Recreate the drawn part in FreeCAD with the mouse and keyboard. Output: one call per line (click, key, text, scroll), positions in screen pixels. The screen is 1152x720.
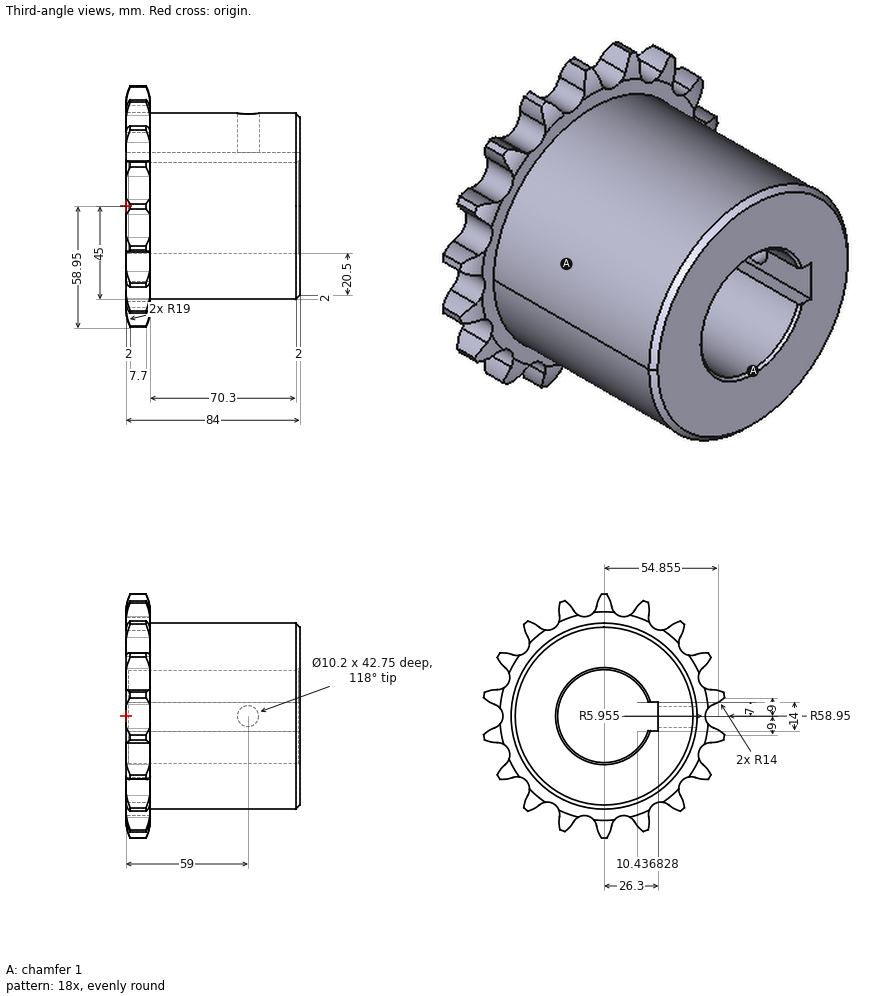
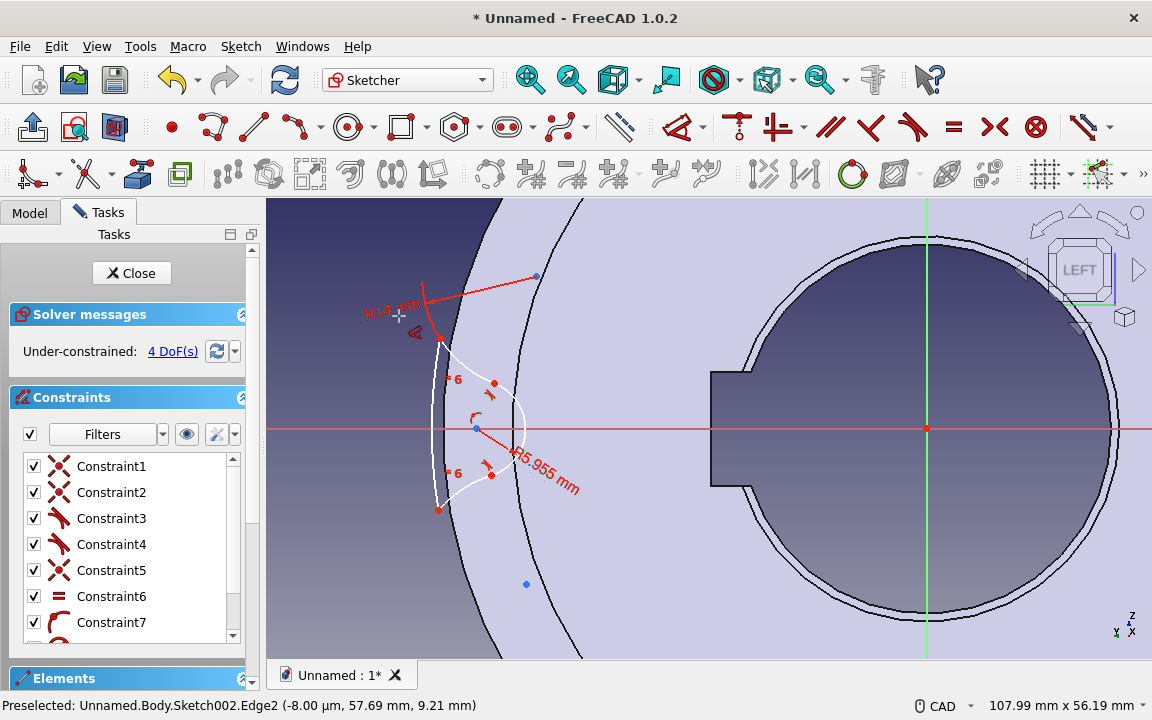
click(433, 390)
click(401, 387)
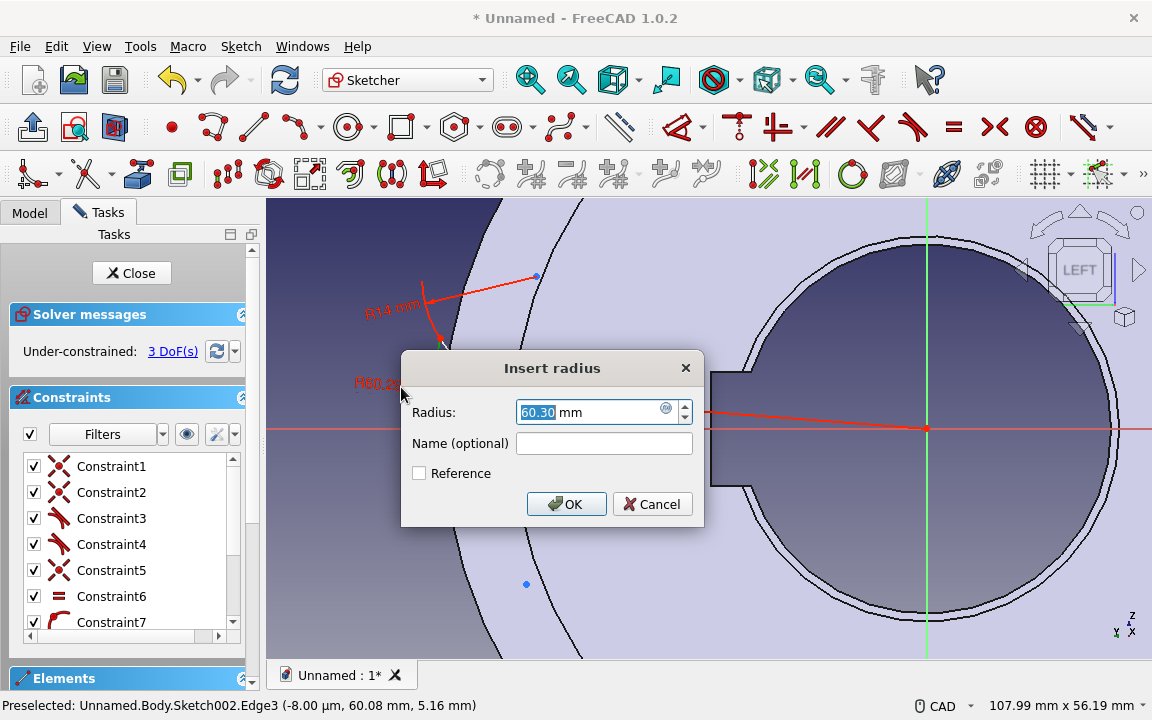
text(58.95)
key(Return)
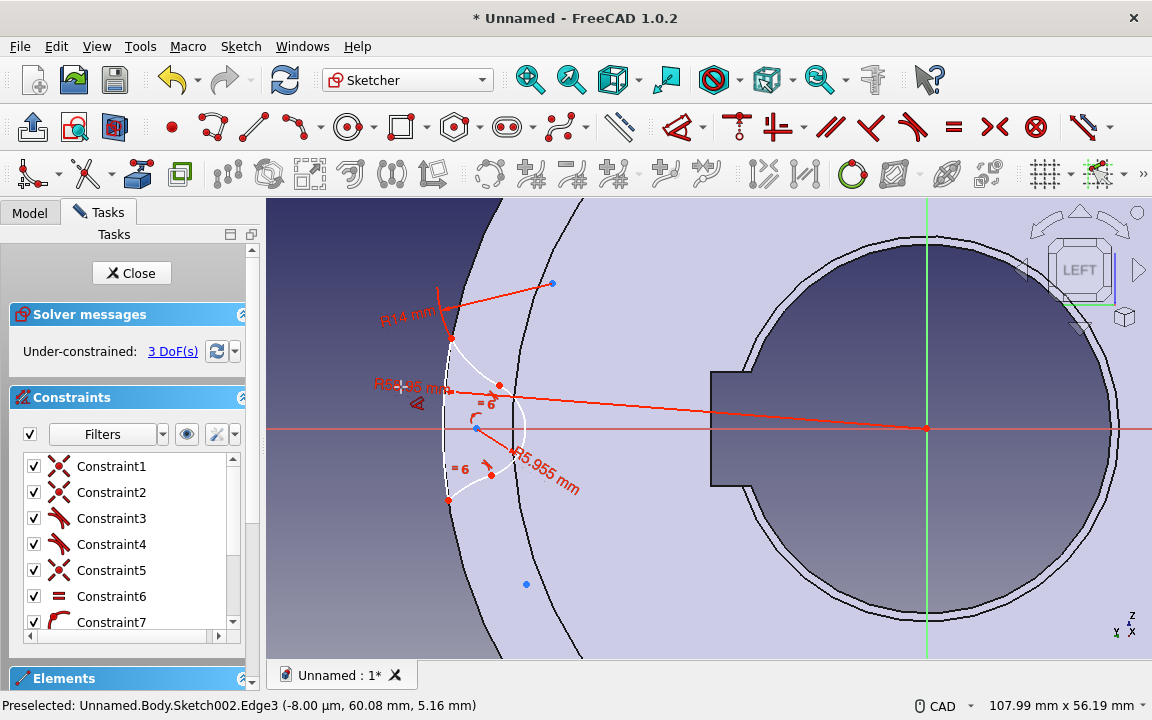
click(451, 339)
click(961, 384)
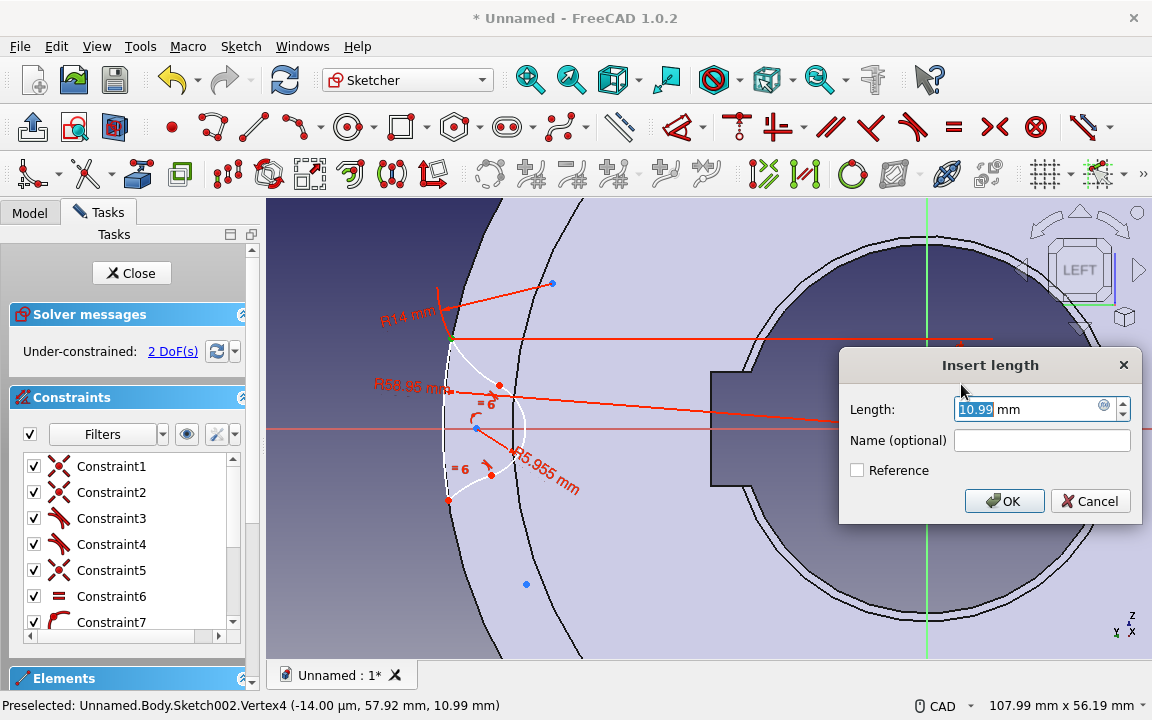
text(9)
key(Return)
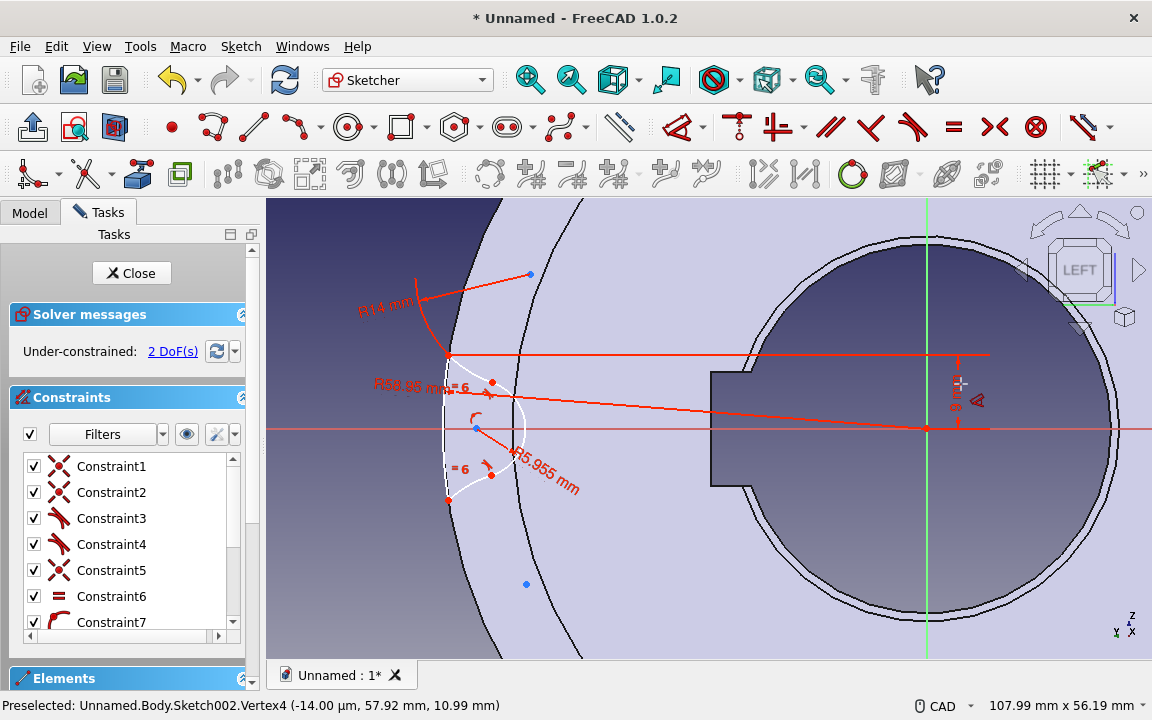
click(448, 501)
click(961, 465)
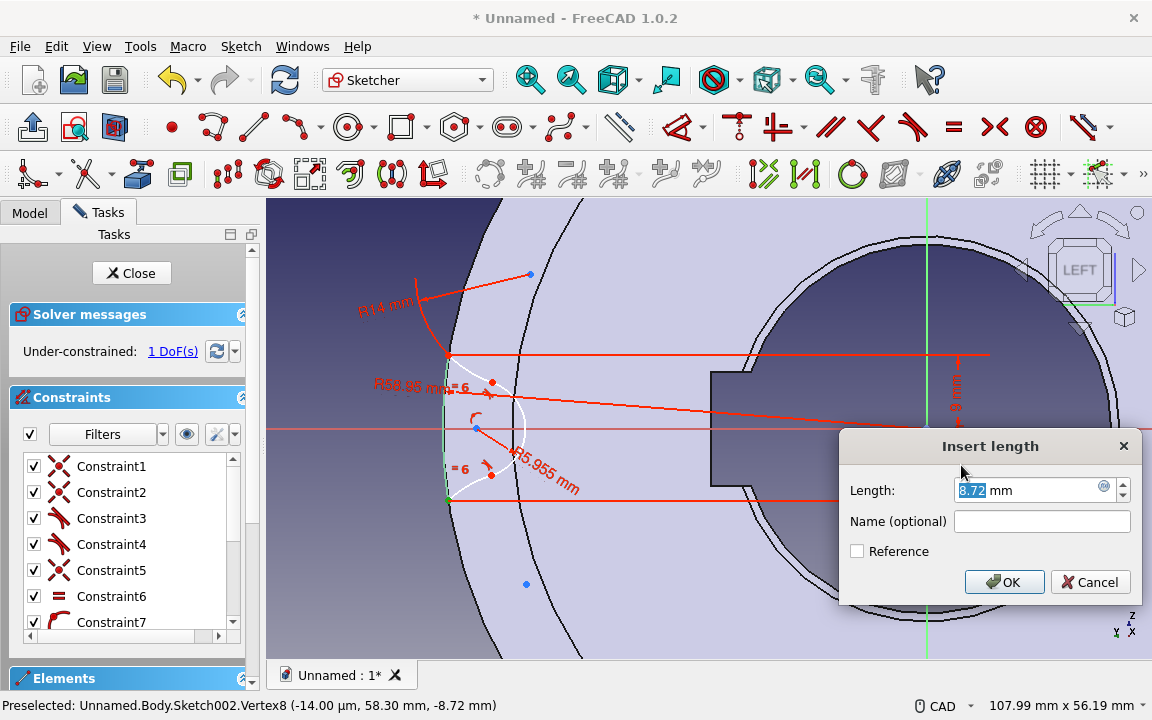
text(9)
key(Return)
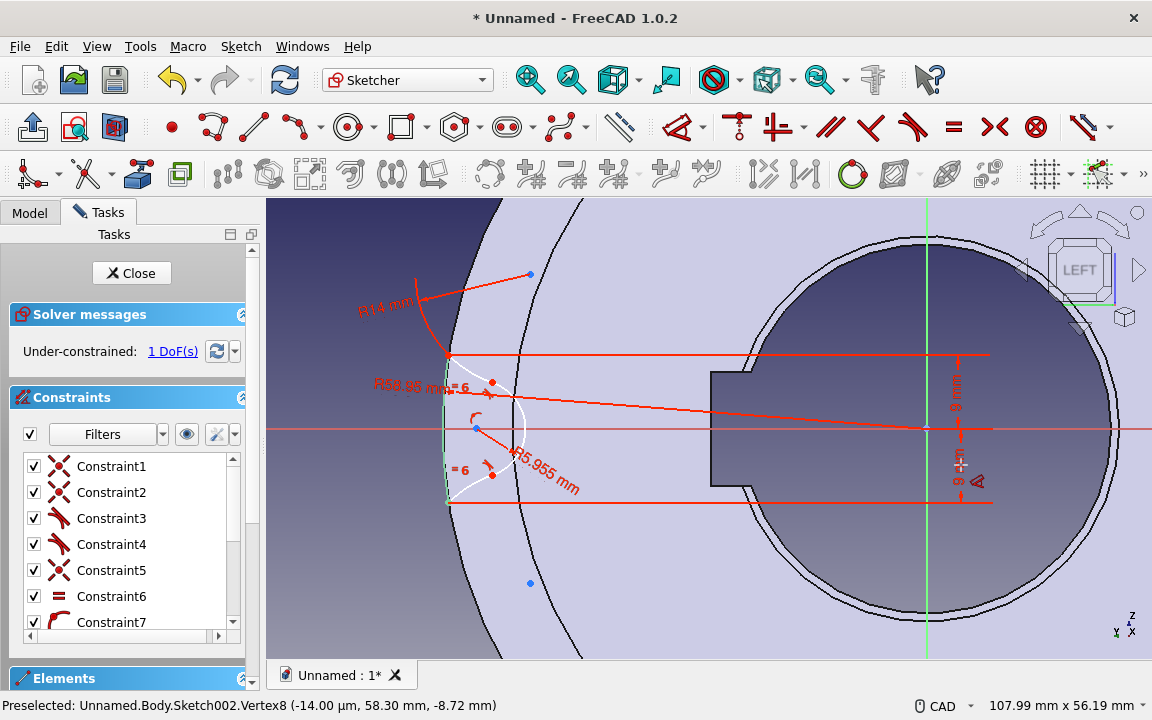
click(477, 429)
click(702, 463)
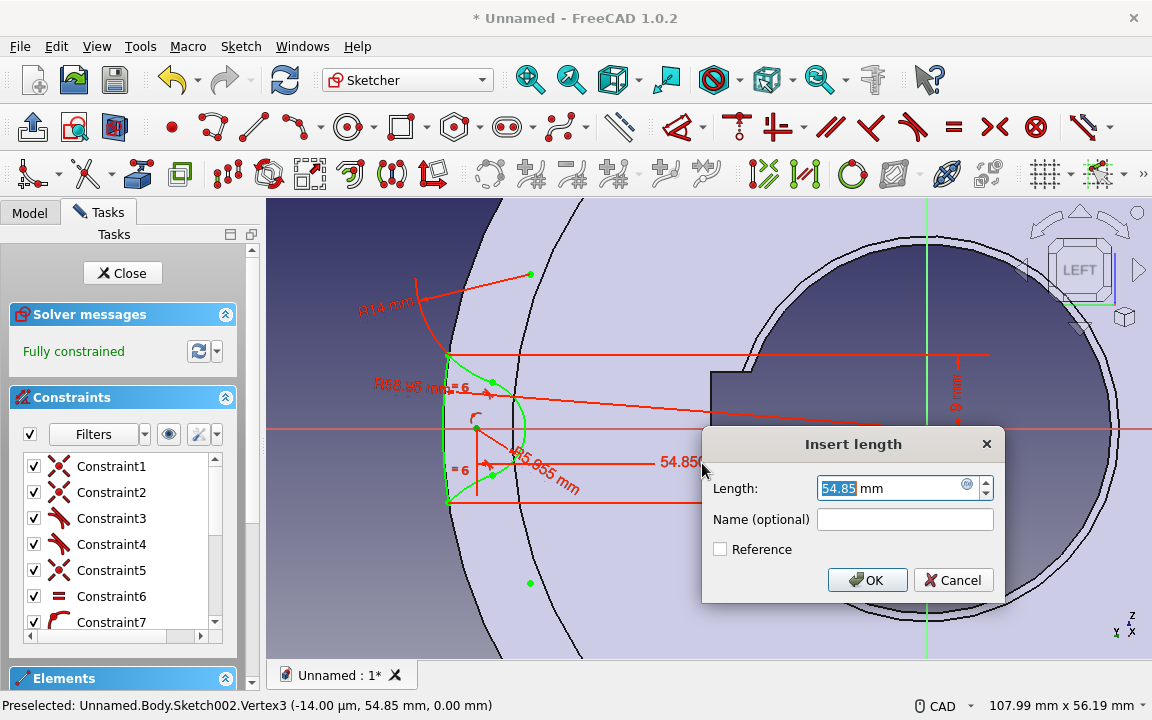
text(54.855)
key(Return)
key(Escape)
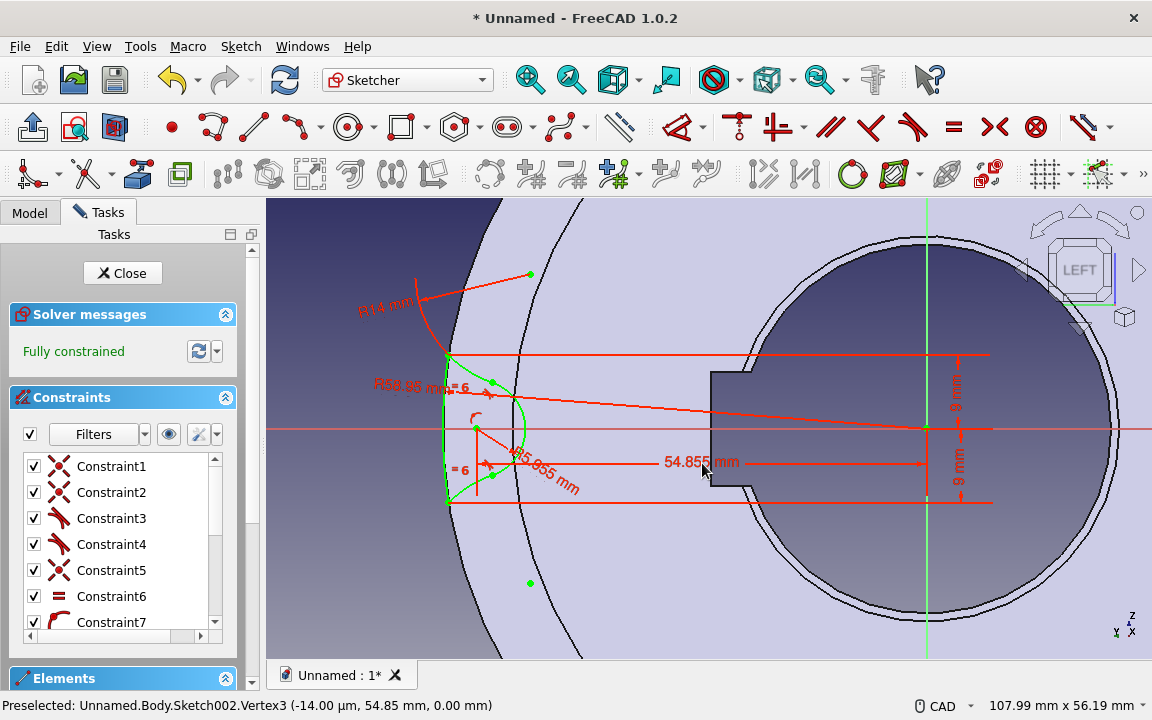
click(123, 273)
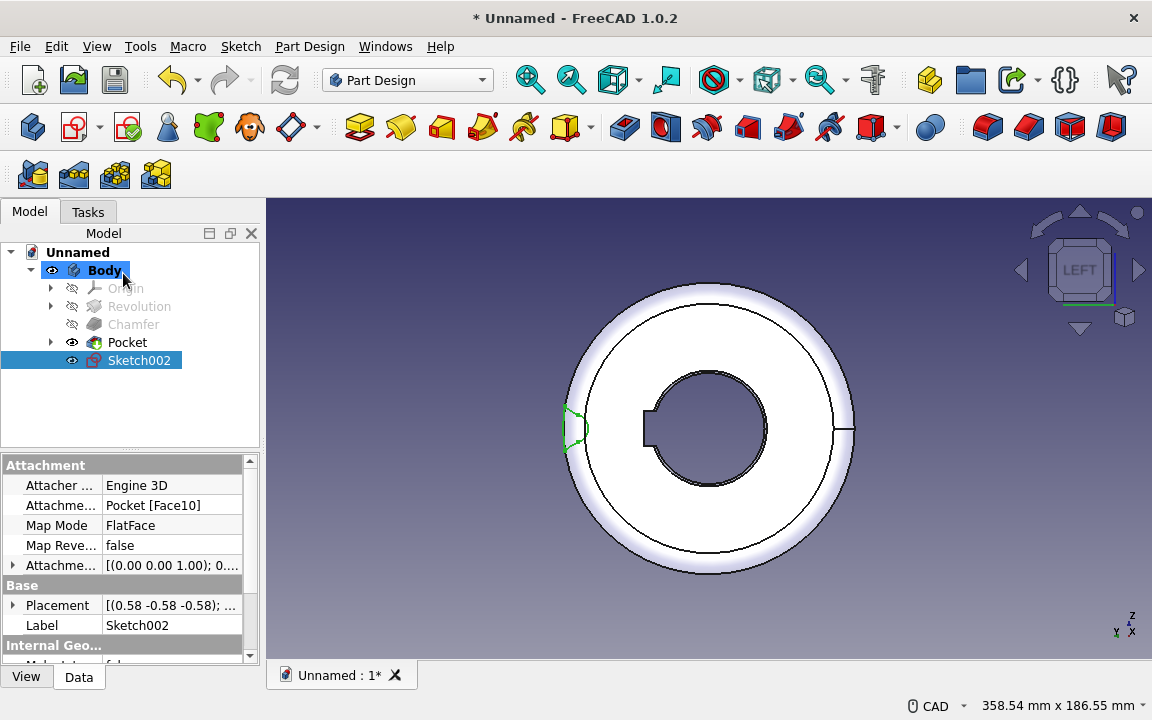
click(625, 128)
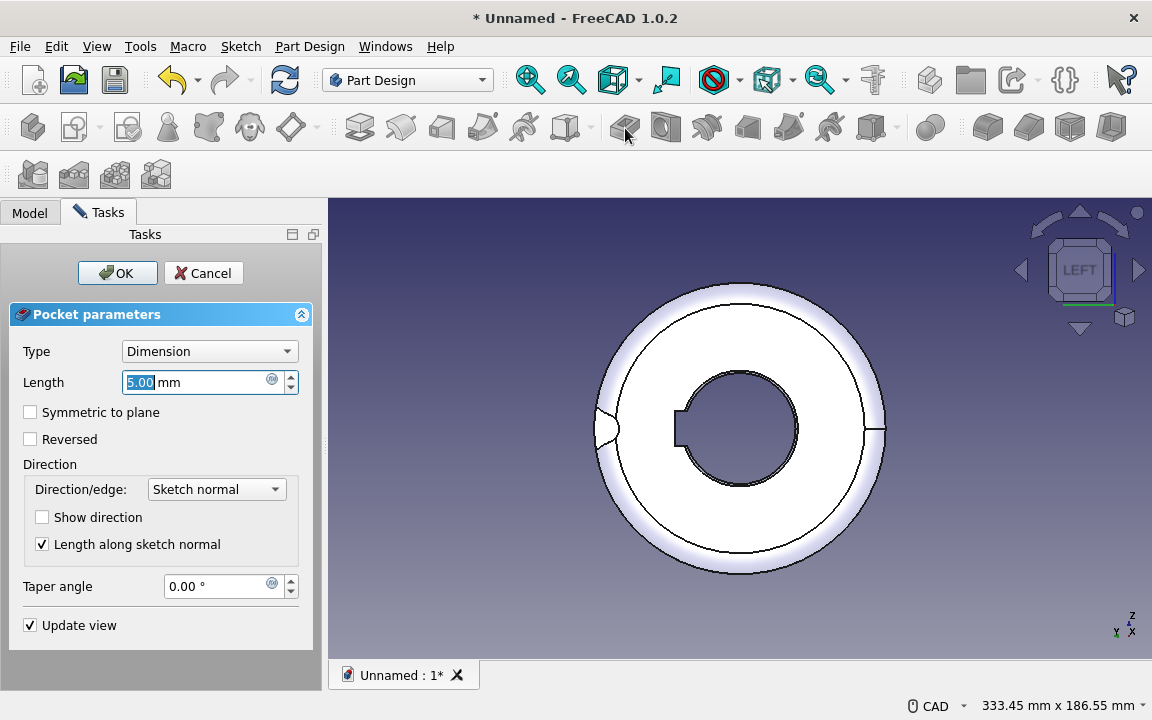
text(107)
key(Tab)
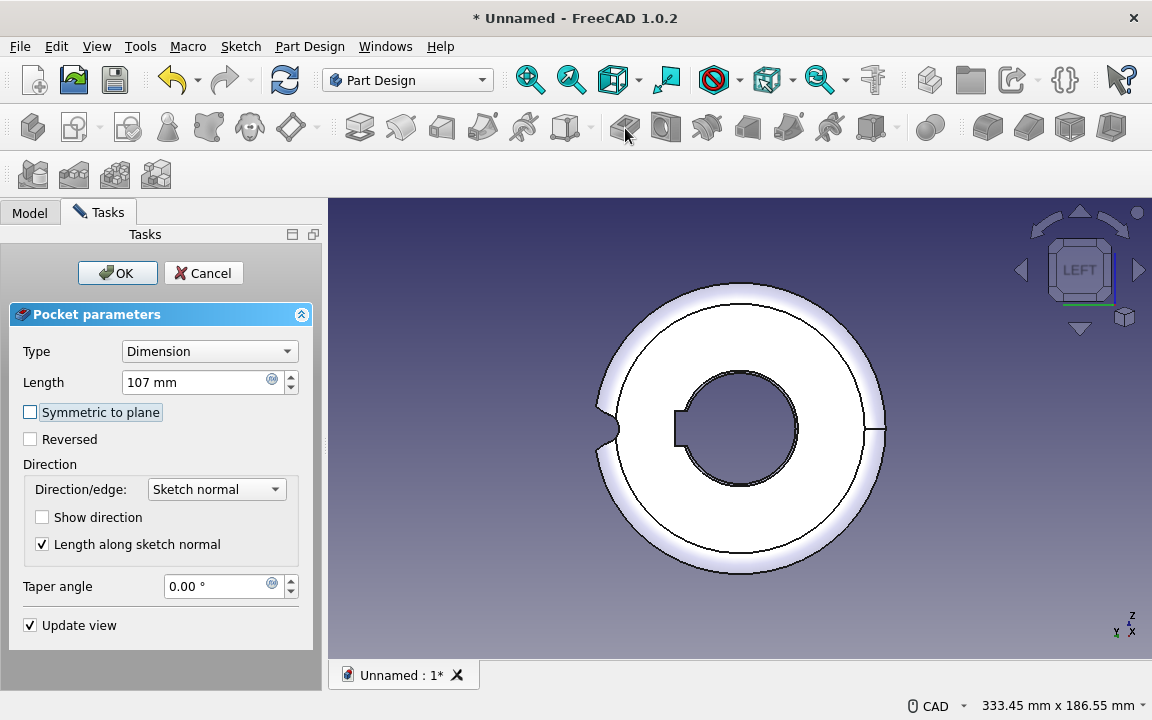
click(118, 273)